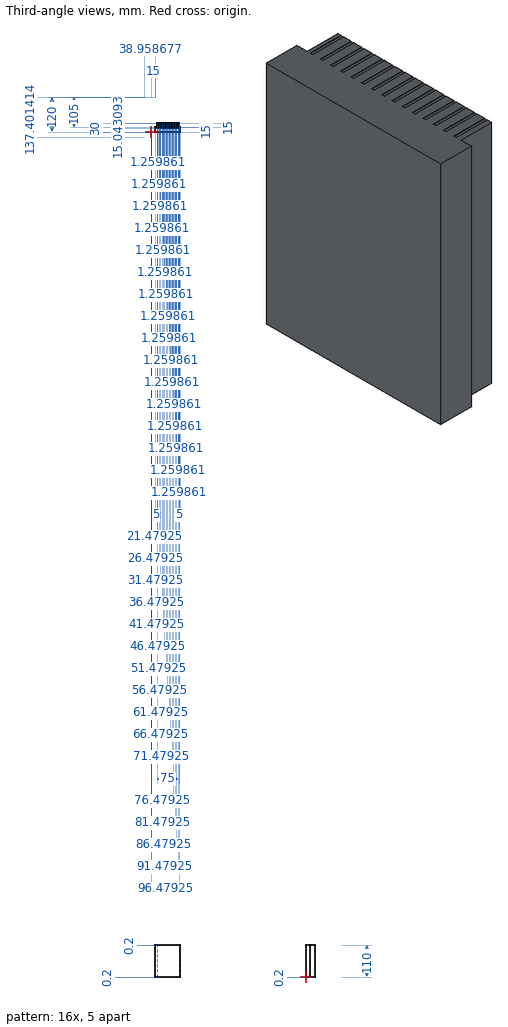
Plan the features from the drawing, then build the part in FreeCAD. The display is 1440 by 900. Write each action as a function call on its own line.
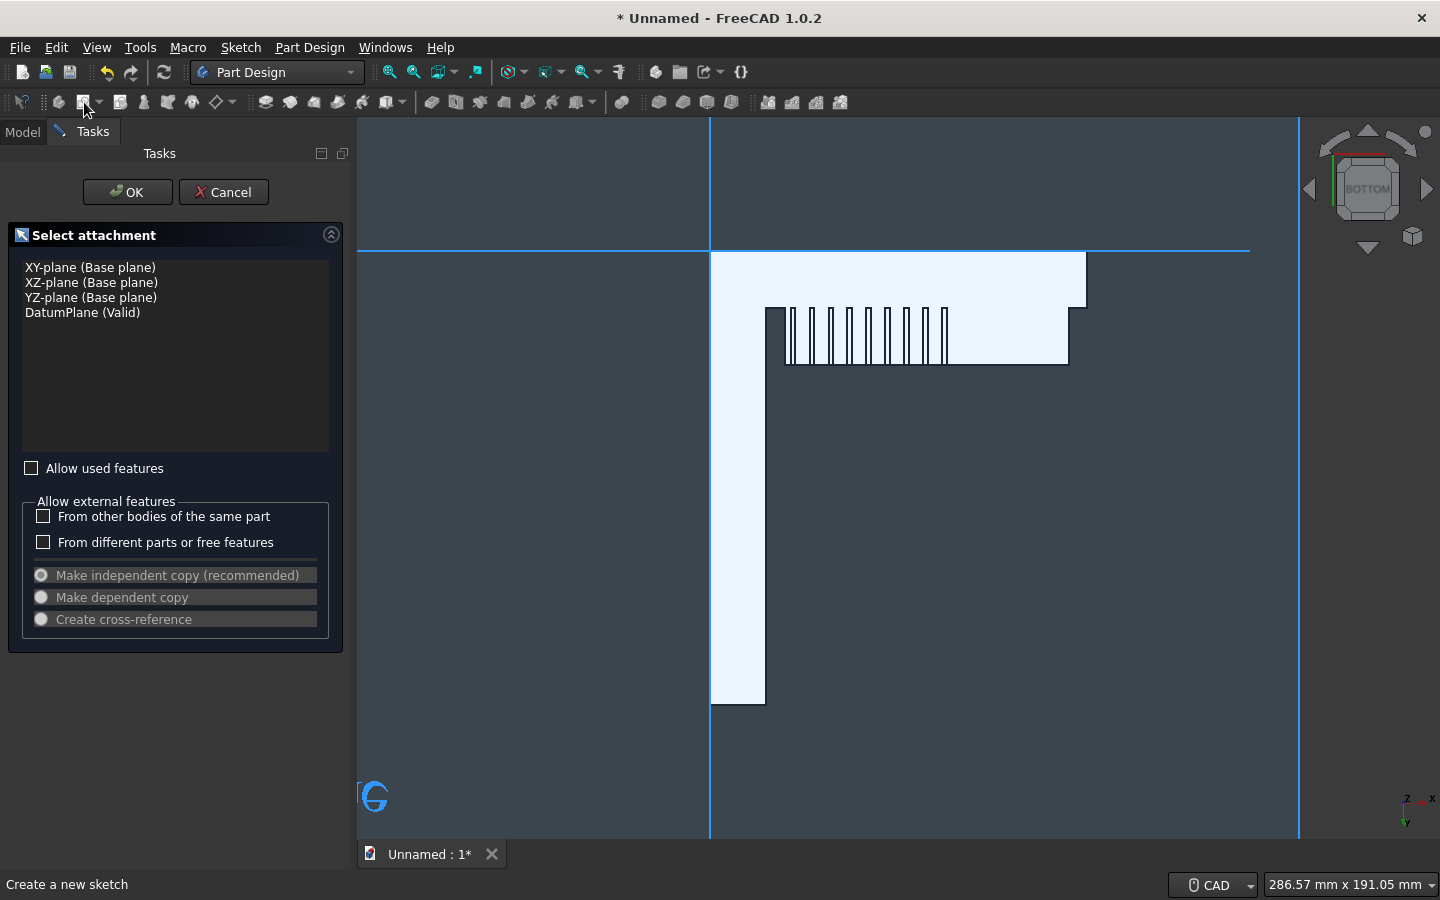
click(82, 268)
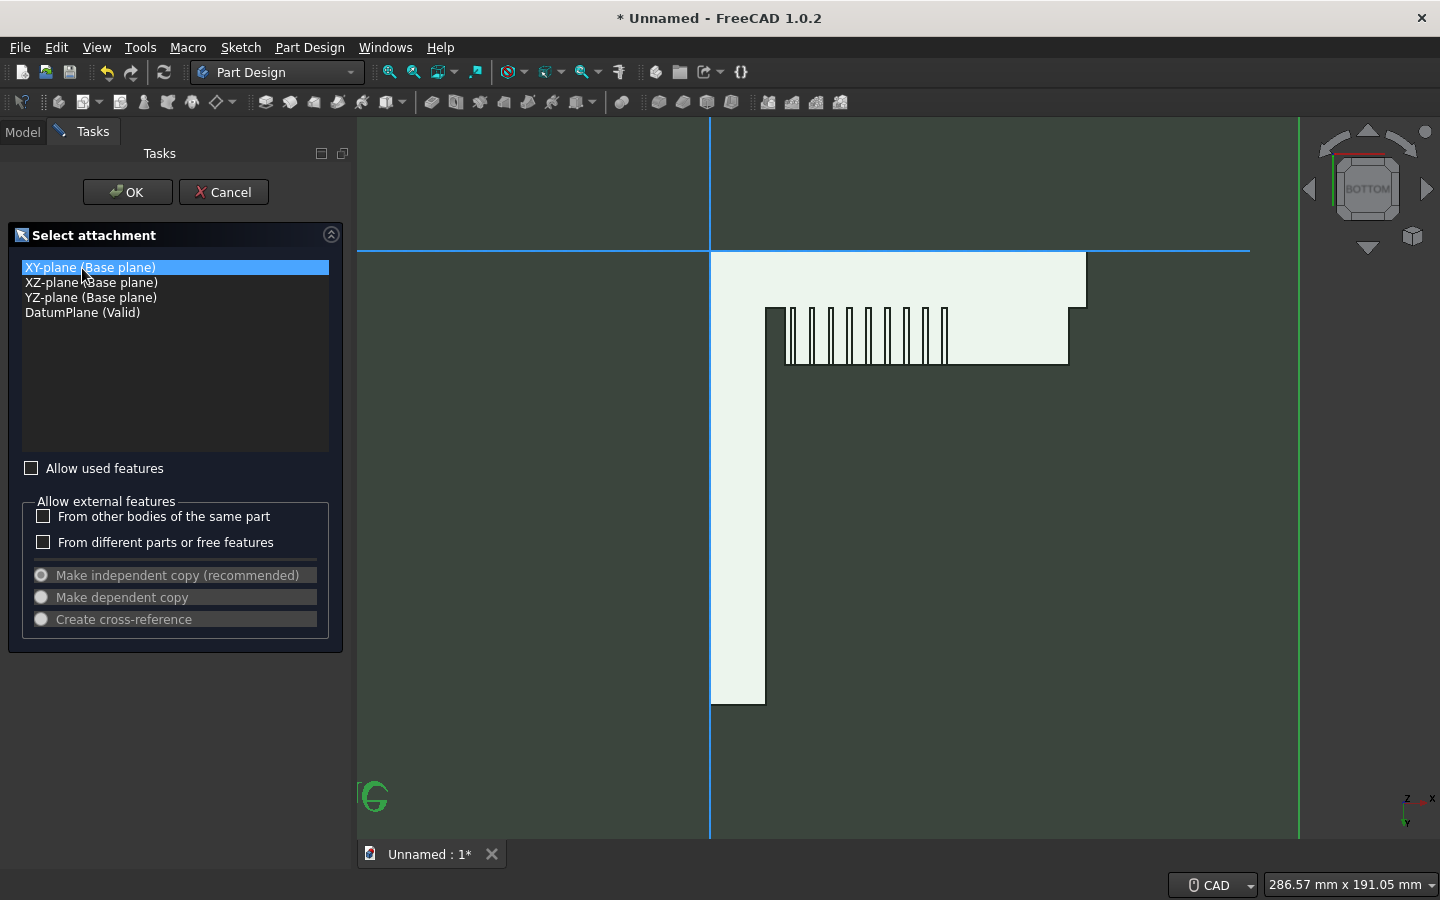
click(128, 192)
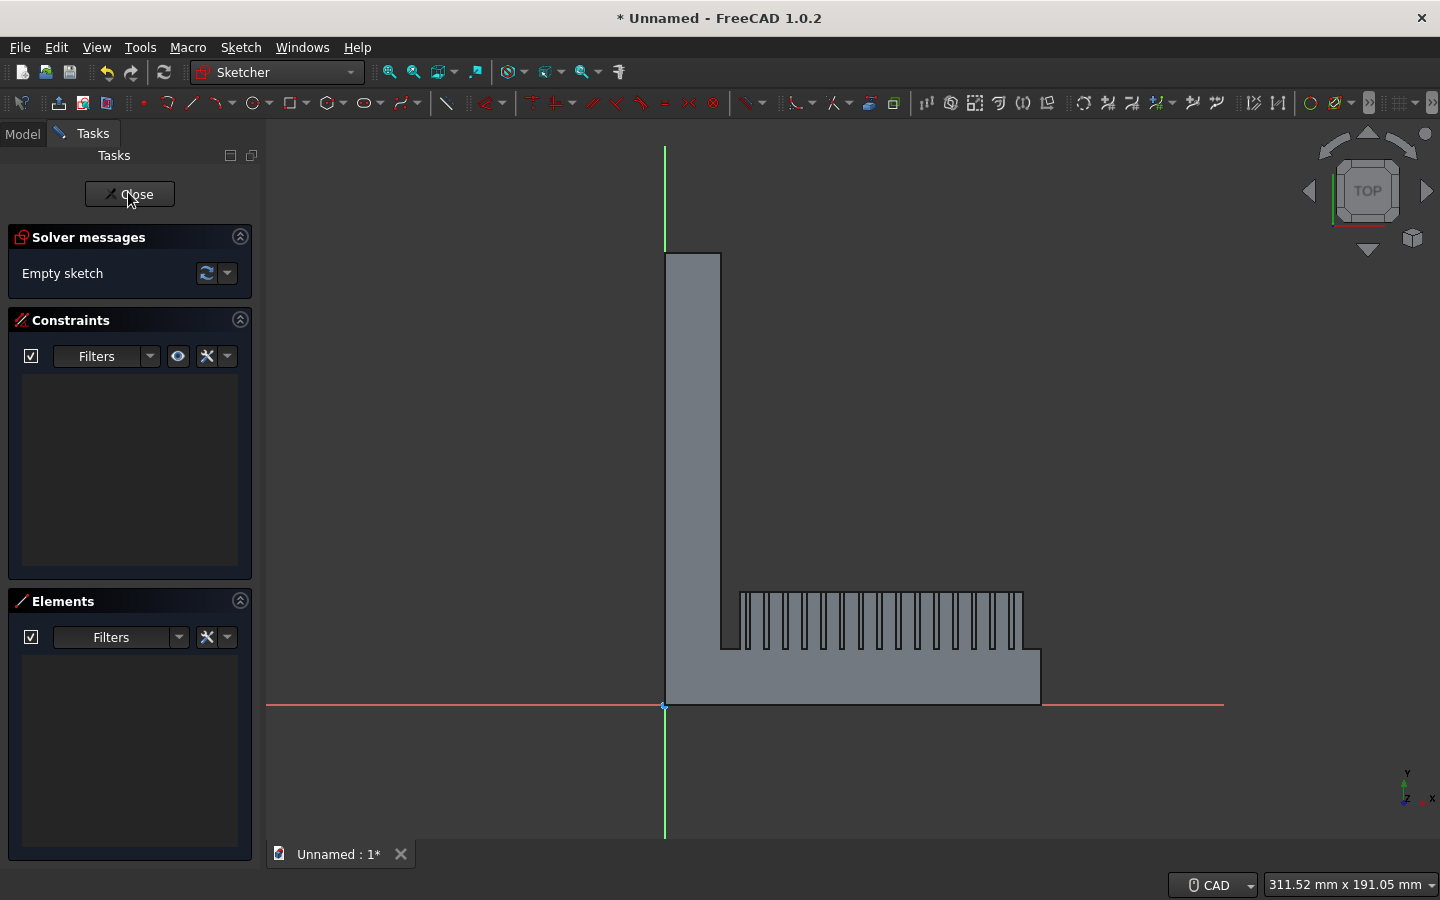
click(108, 104)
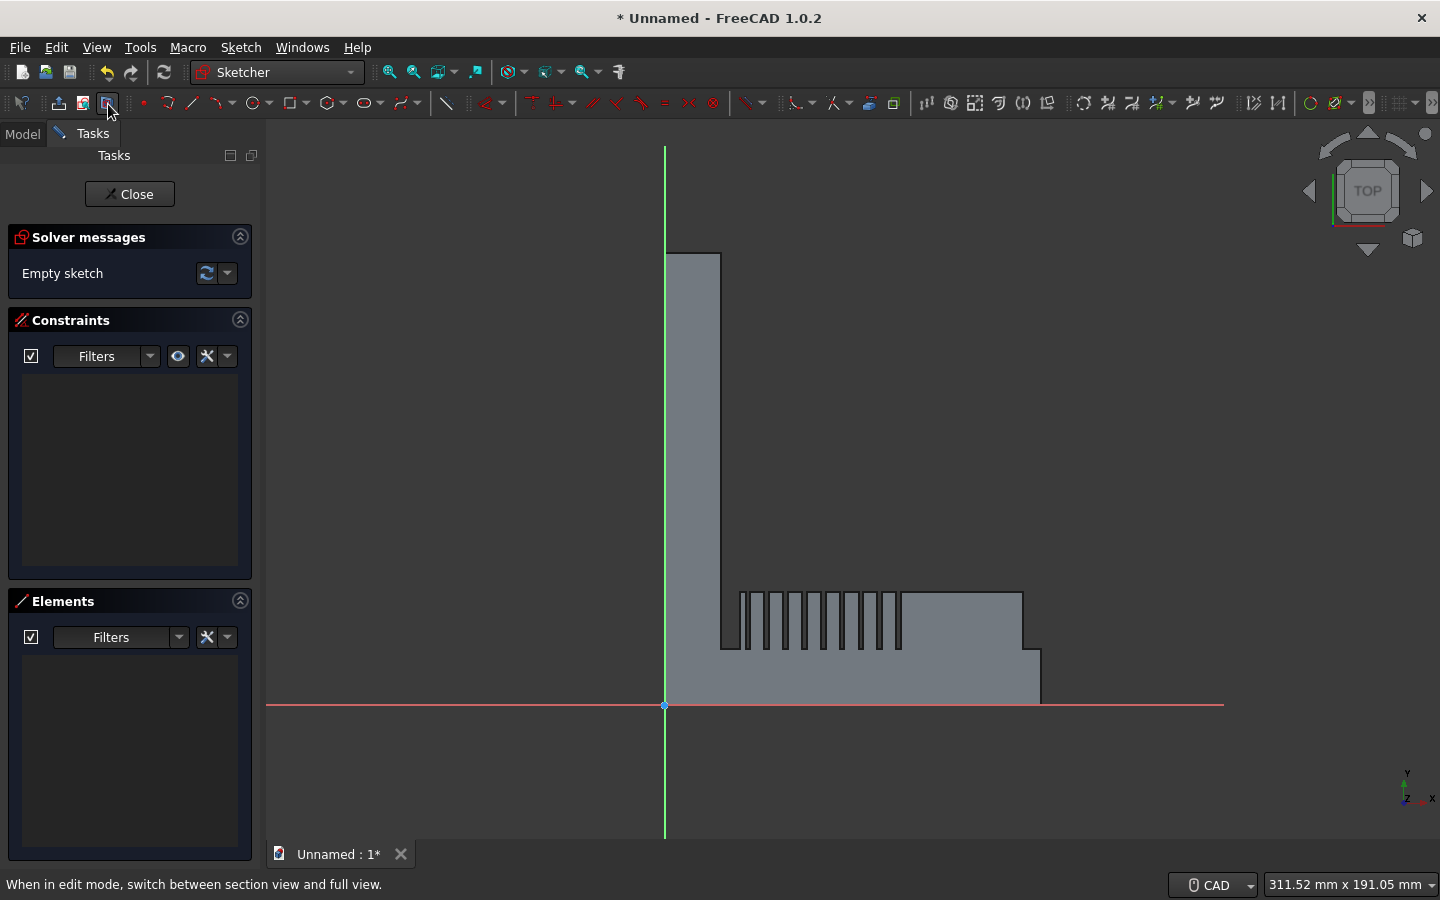
scroll(934, 638, up, 11)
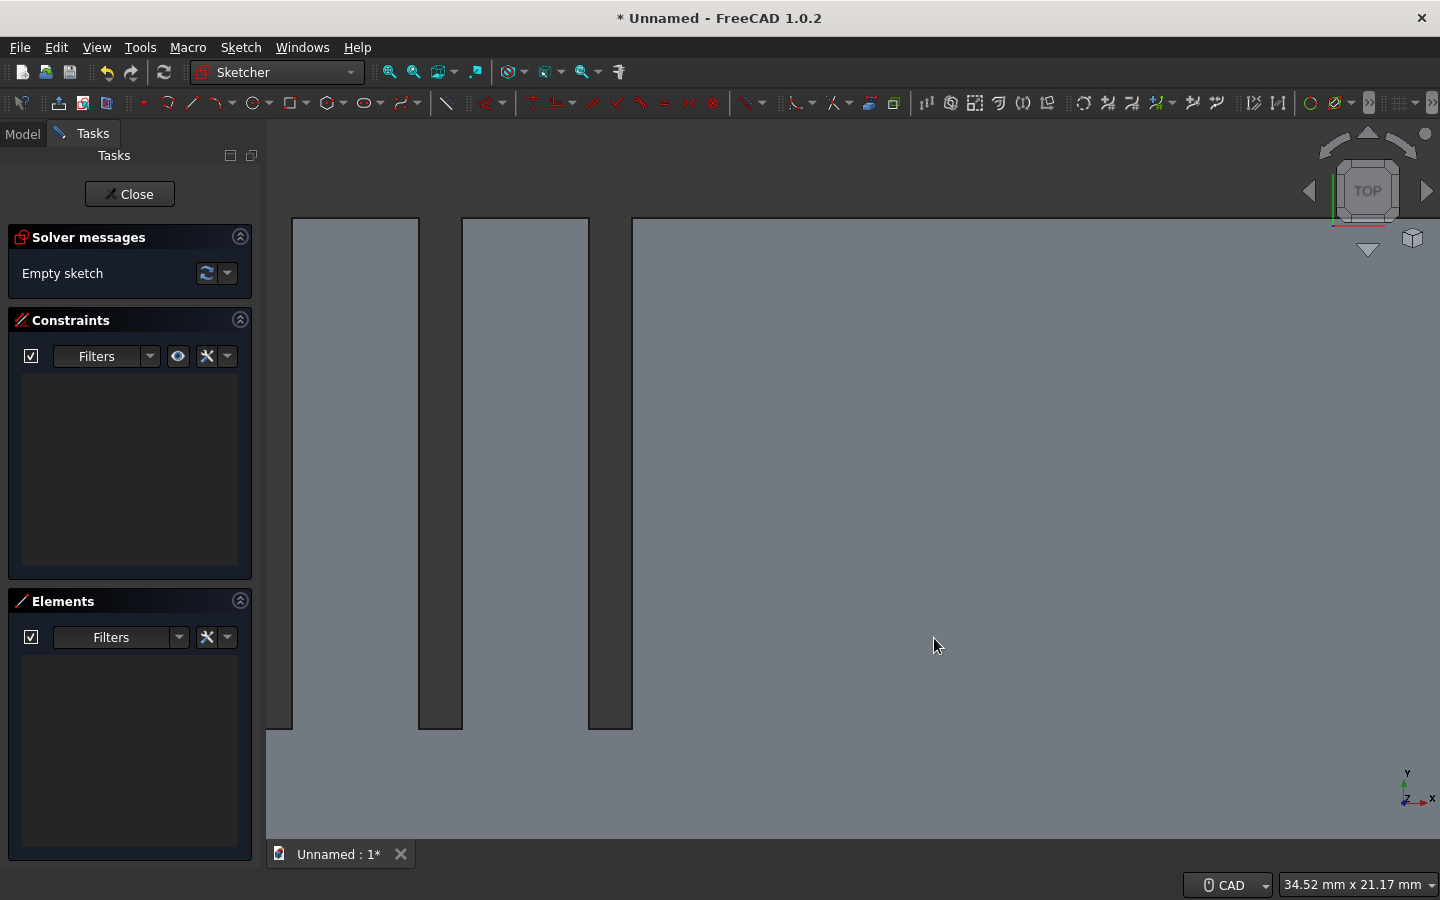
click(290, 104)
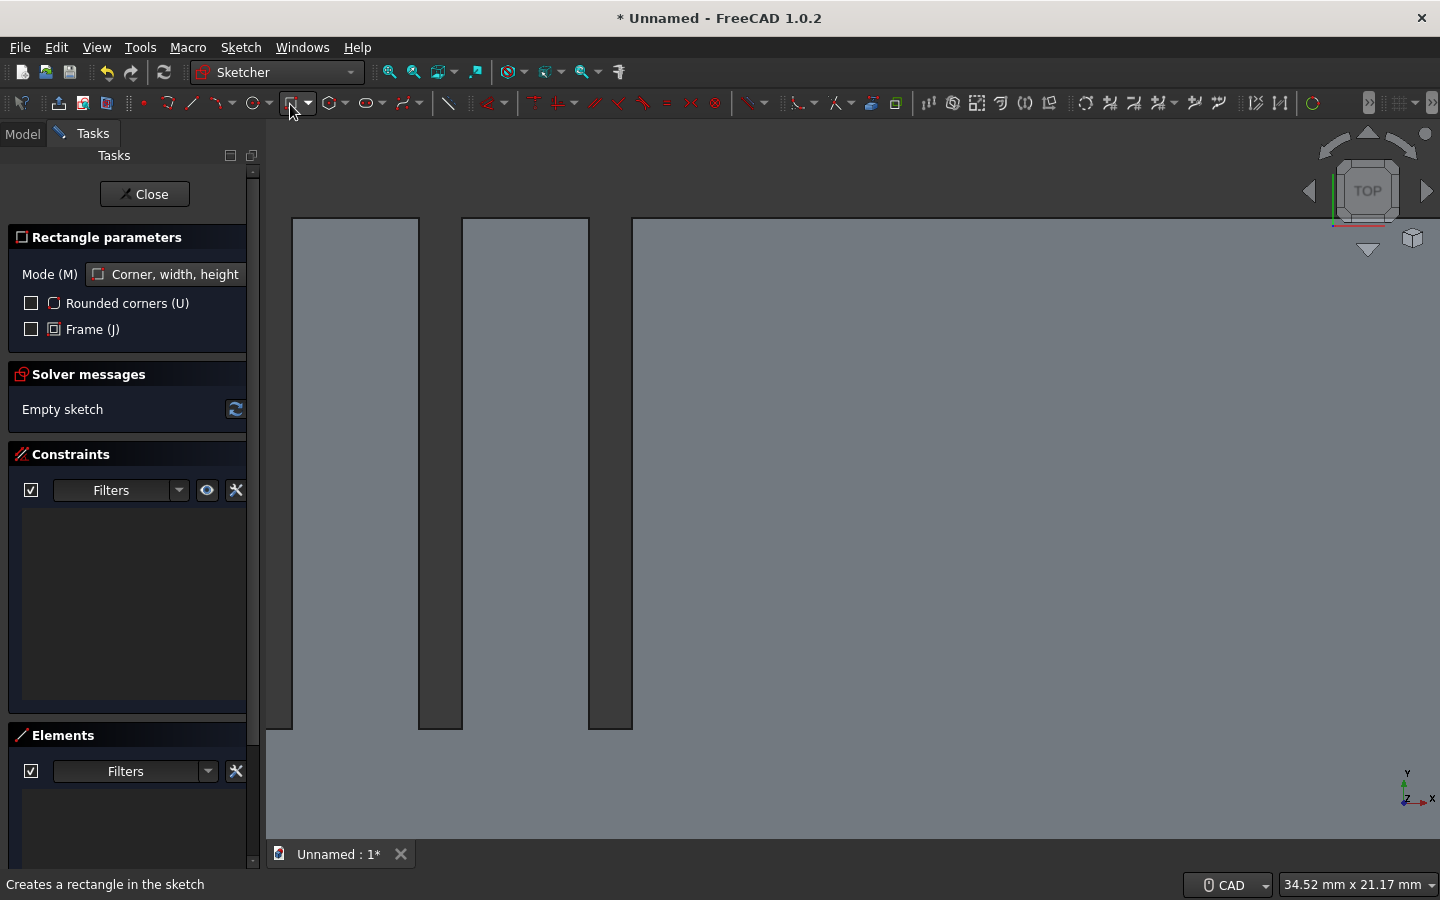
click(759, 218)
click(802, 729)
key(Escape)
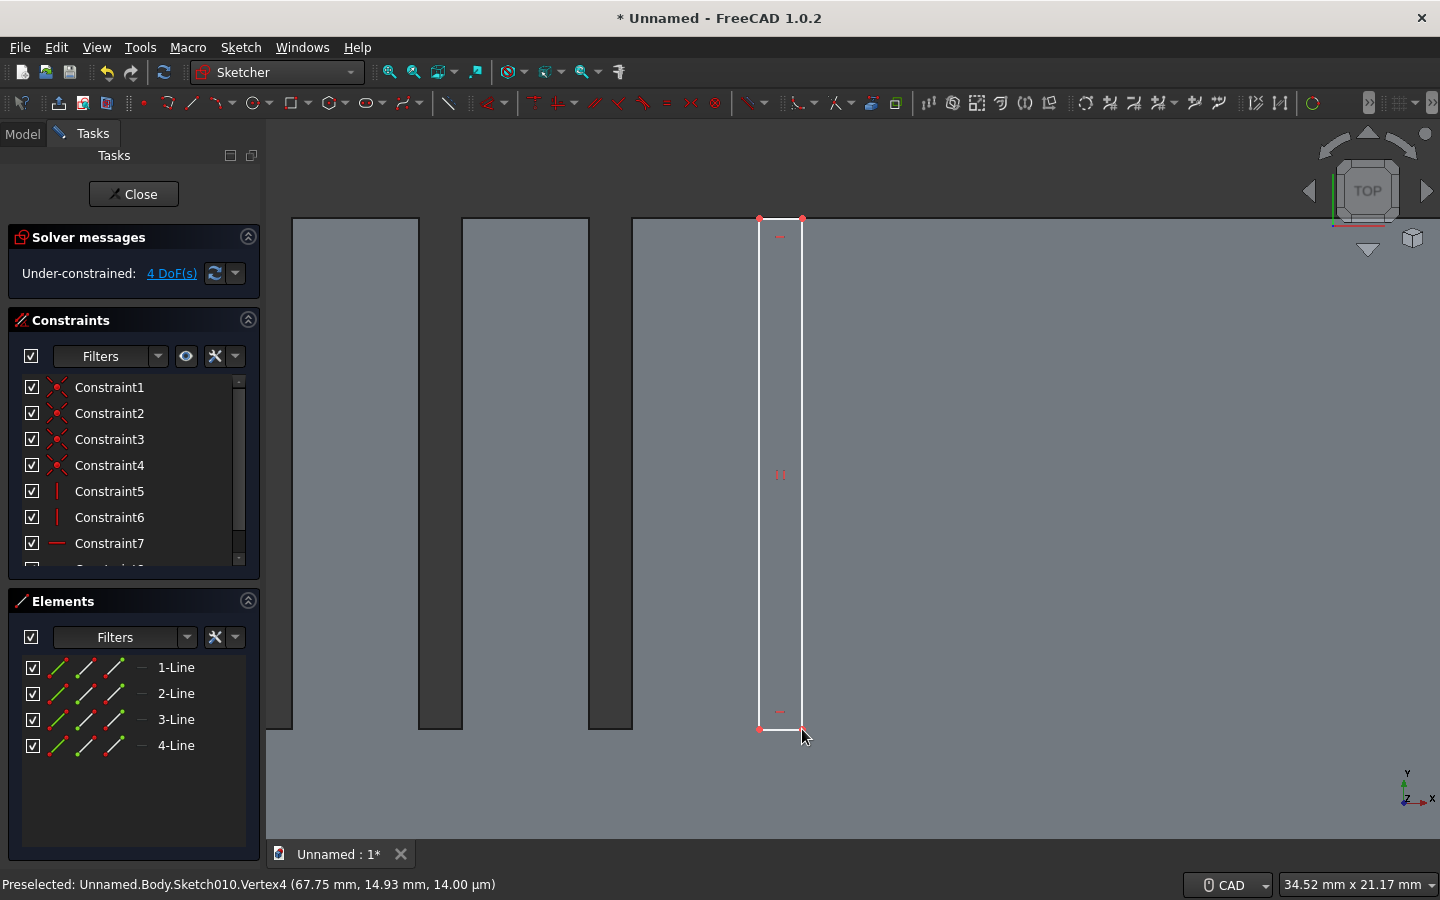
click(488, 104)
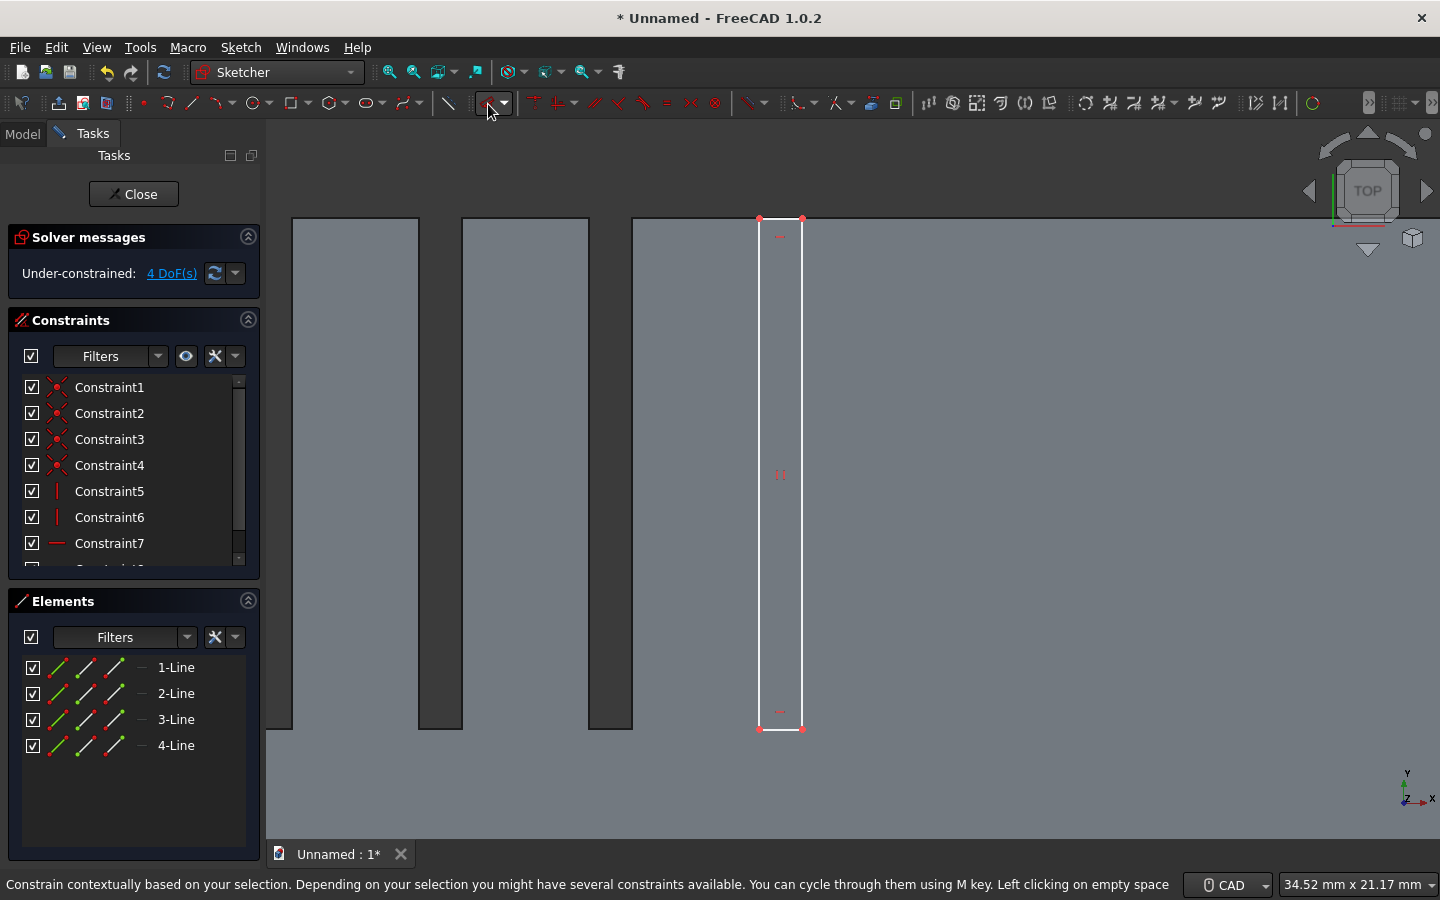
click(759, 219)
click(817, 515)